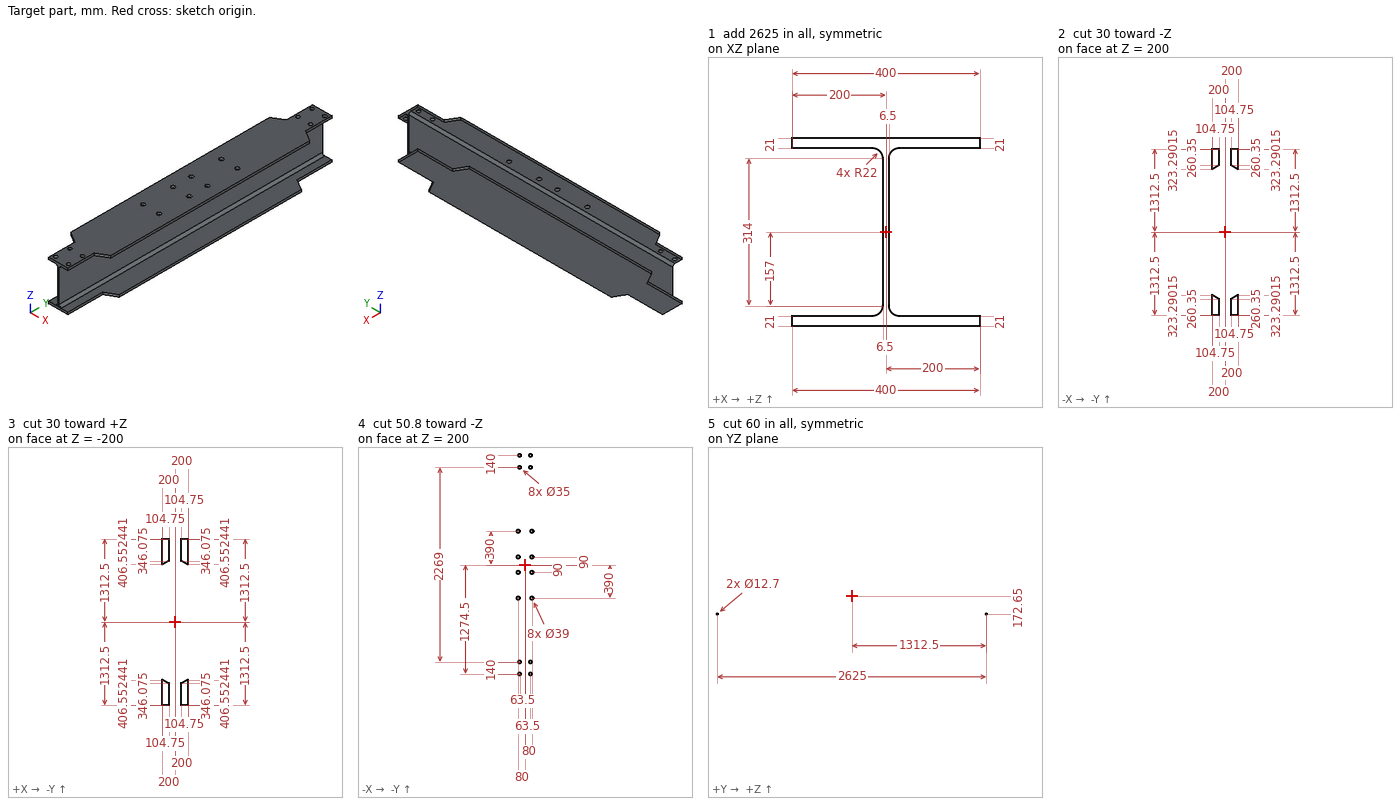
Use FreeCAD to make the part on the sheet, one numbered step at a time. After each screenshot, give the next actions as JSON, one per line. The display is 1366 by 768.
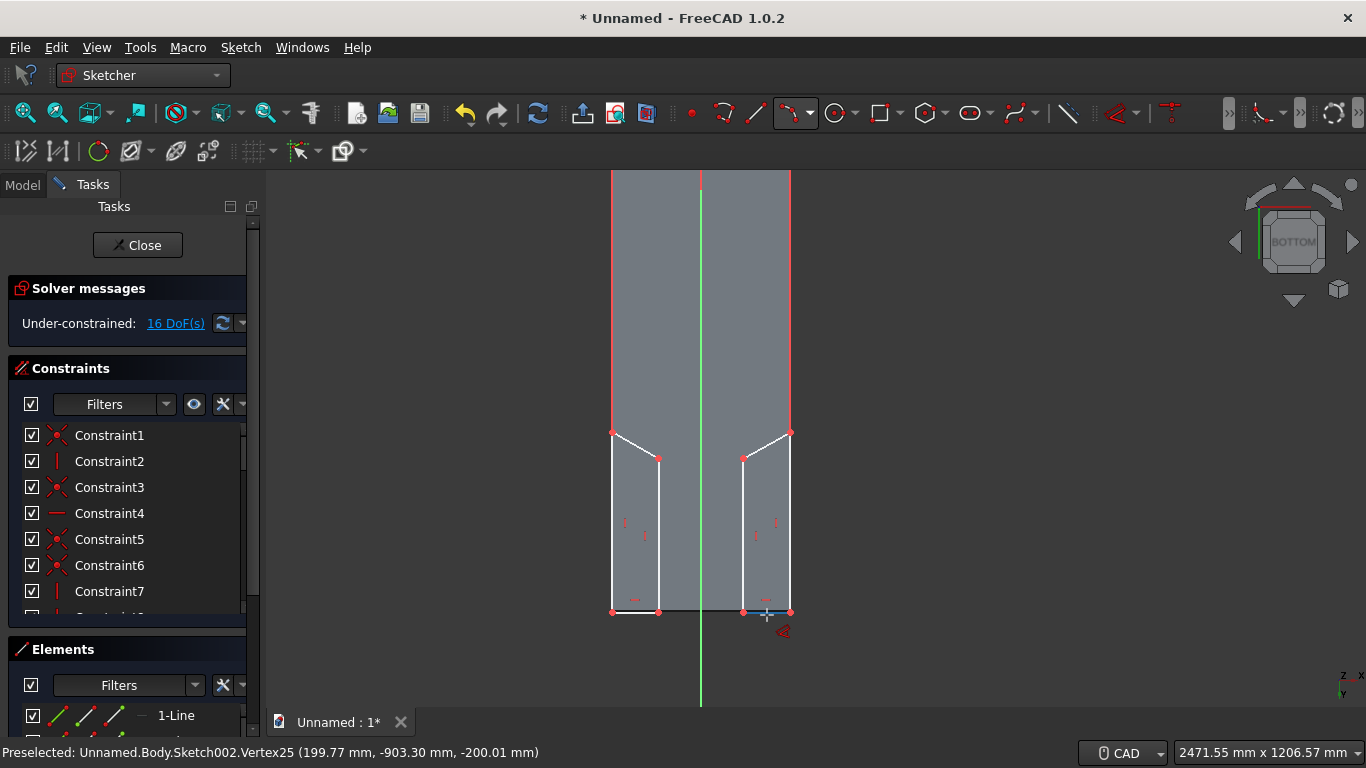
{"action": "left_click", "coordinate": [767, 613]}
{"action": "left_click", "coordinate": [767, 647]}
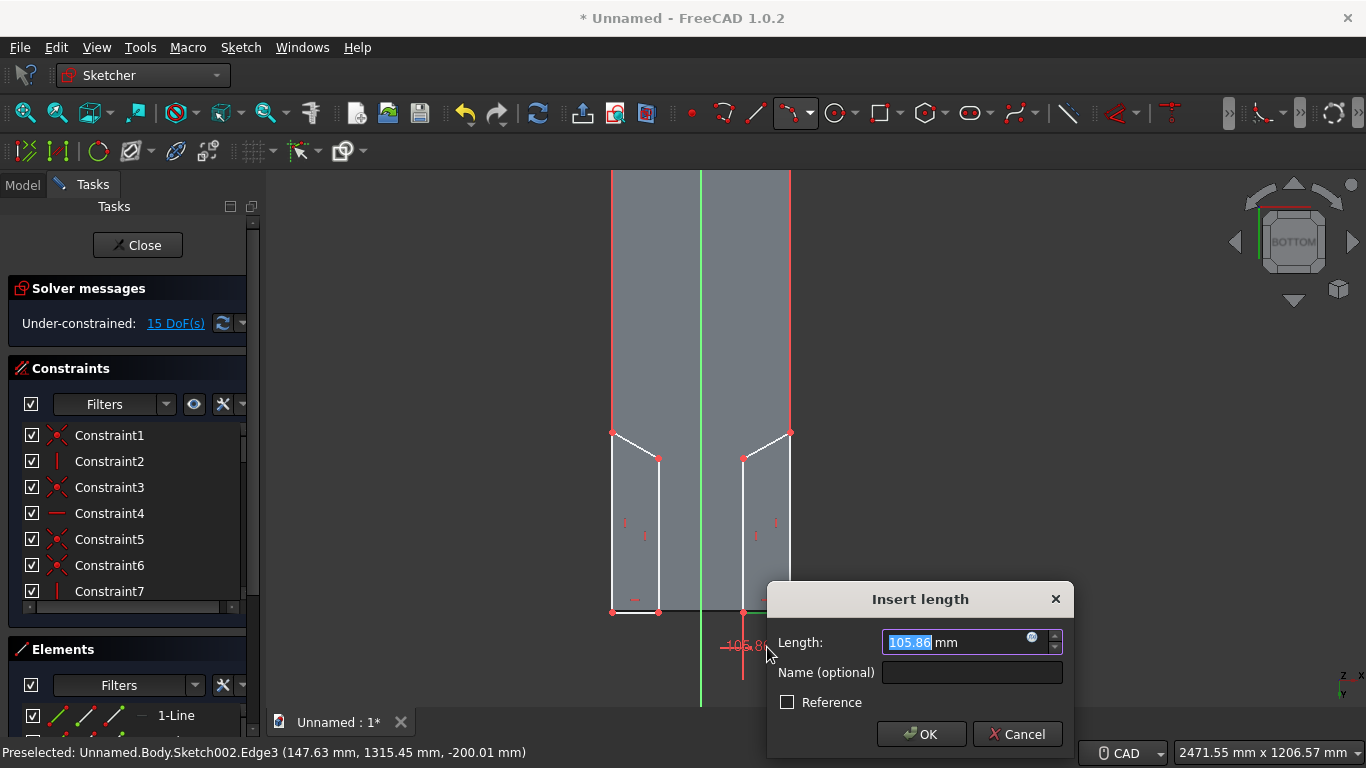
{"action": "type", "text": "104.75"}
{"action": "key", "text": "Return"}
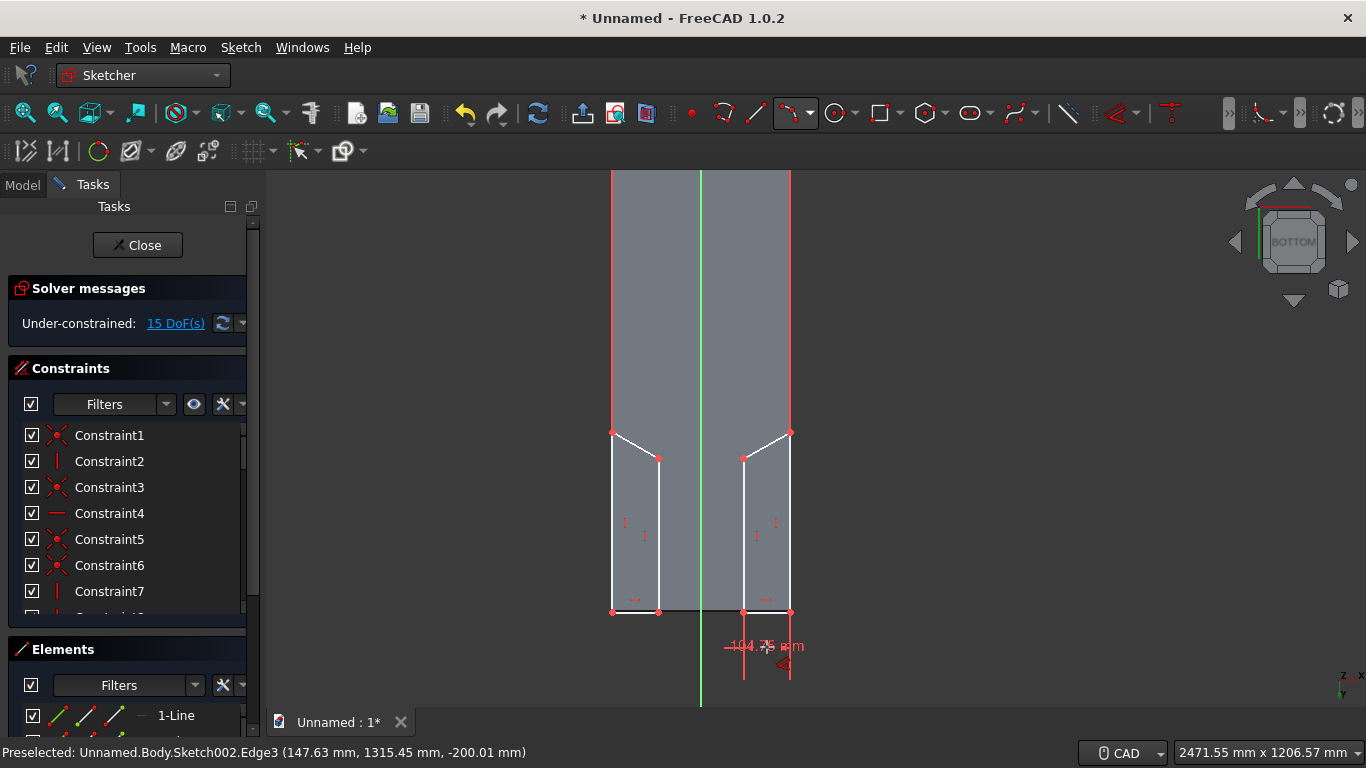
{"action": "left_click", "coordinate": [626, 613]}
{"action": "left_click", "coordinate": [636, 647]}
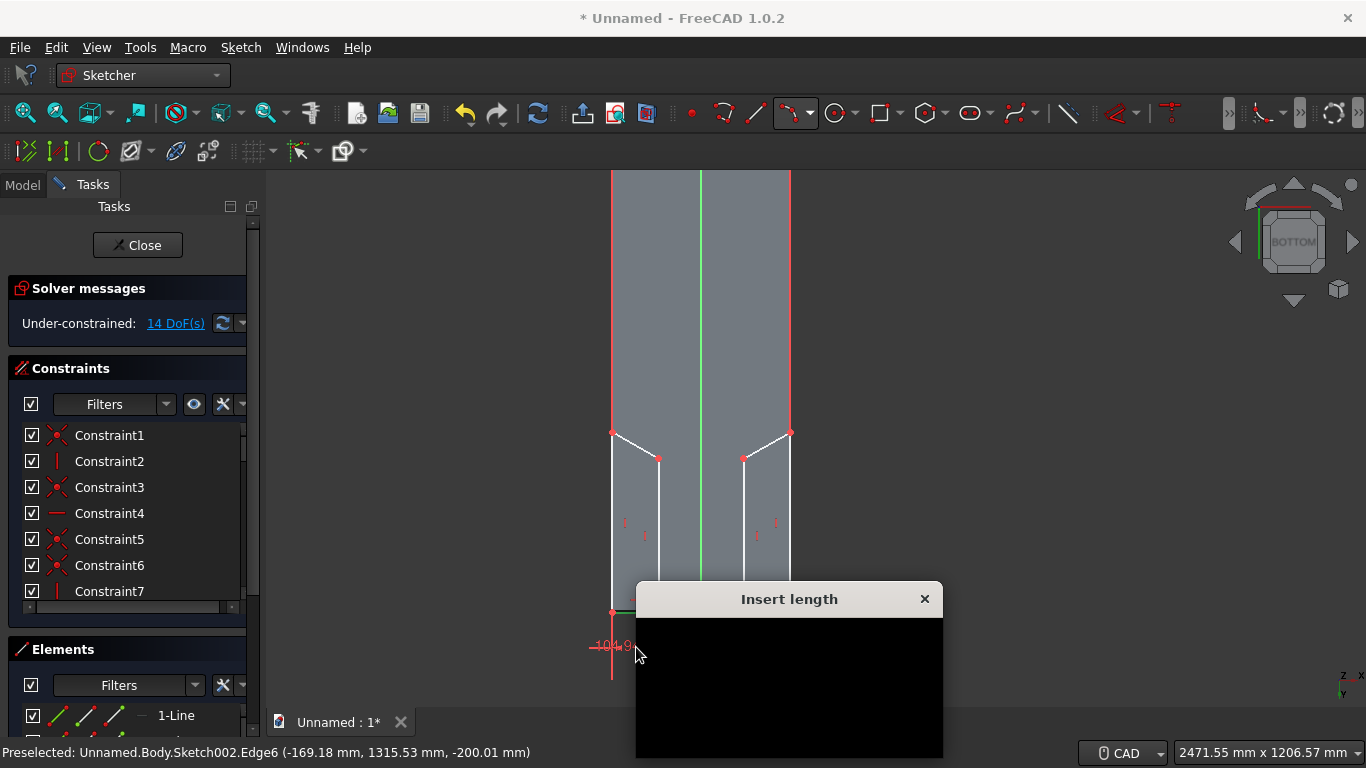
{"action": "type", "text": "104.75"}
{"action": "key", "text": "Return"}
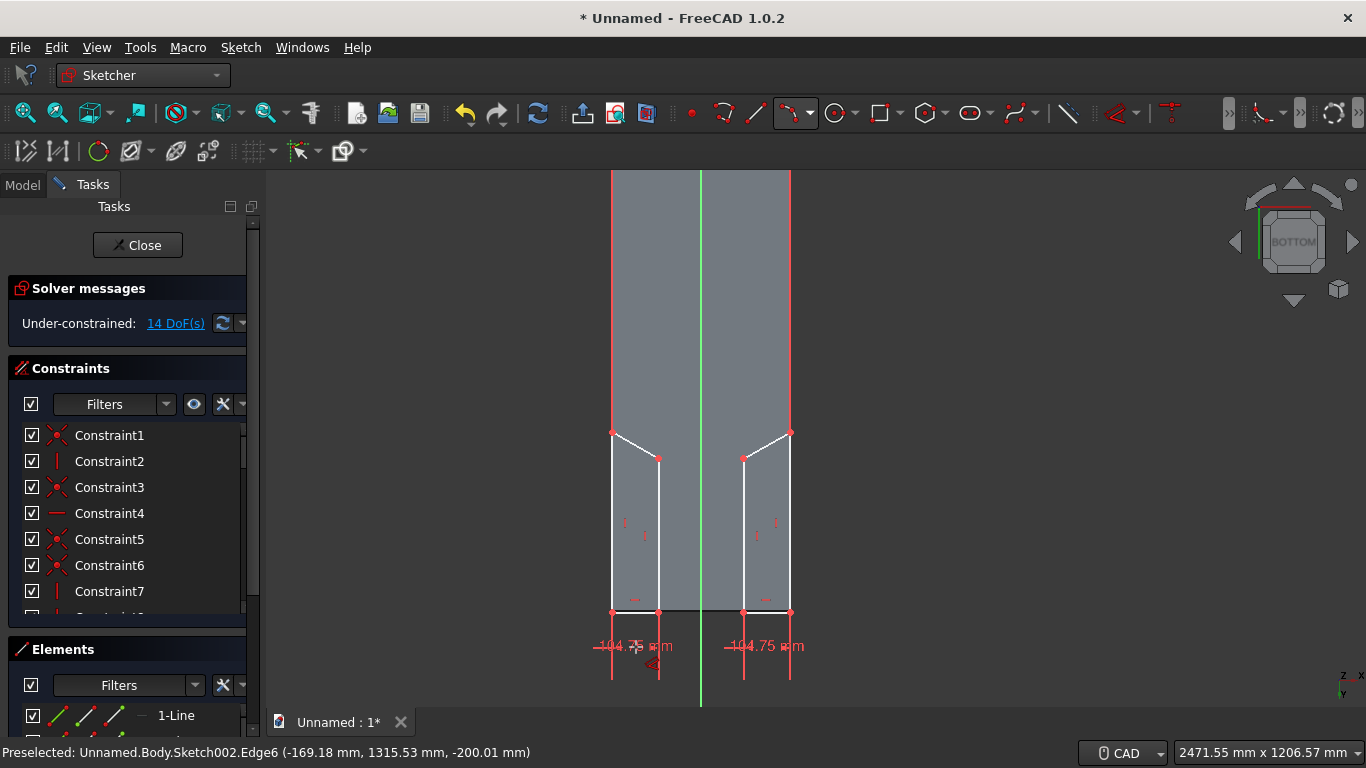
{"action": "scroll", "coordinate": [767, 616], "scroll_direction": "down", "scroll_amount": 6}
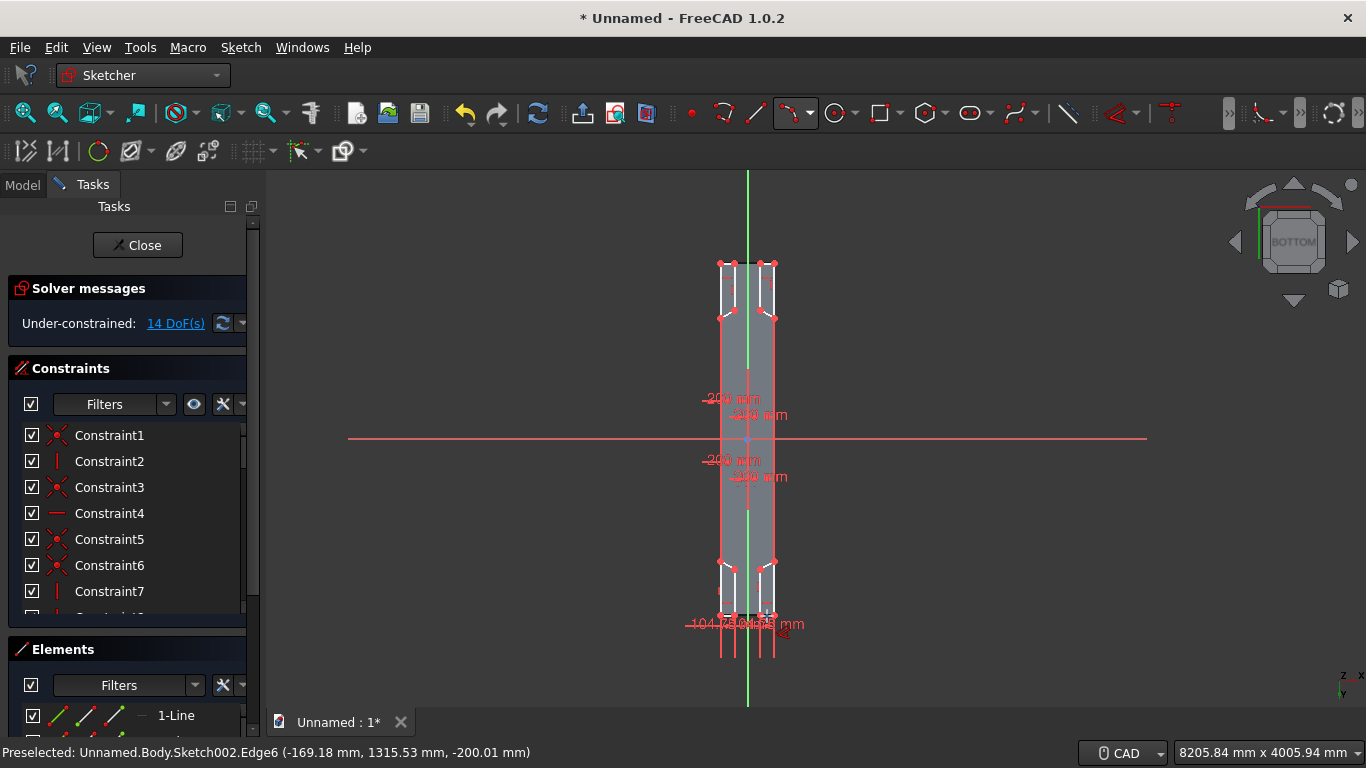
{"action": "scroll", "coordinate": [731, 264], "scroll_direction": "up", "scroll_amount": 6}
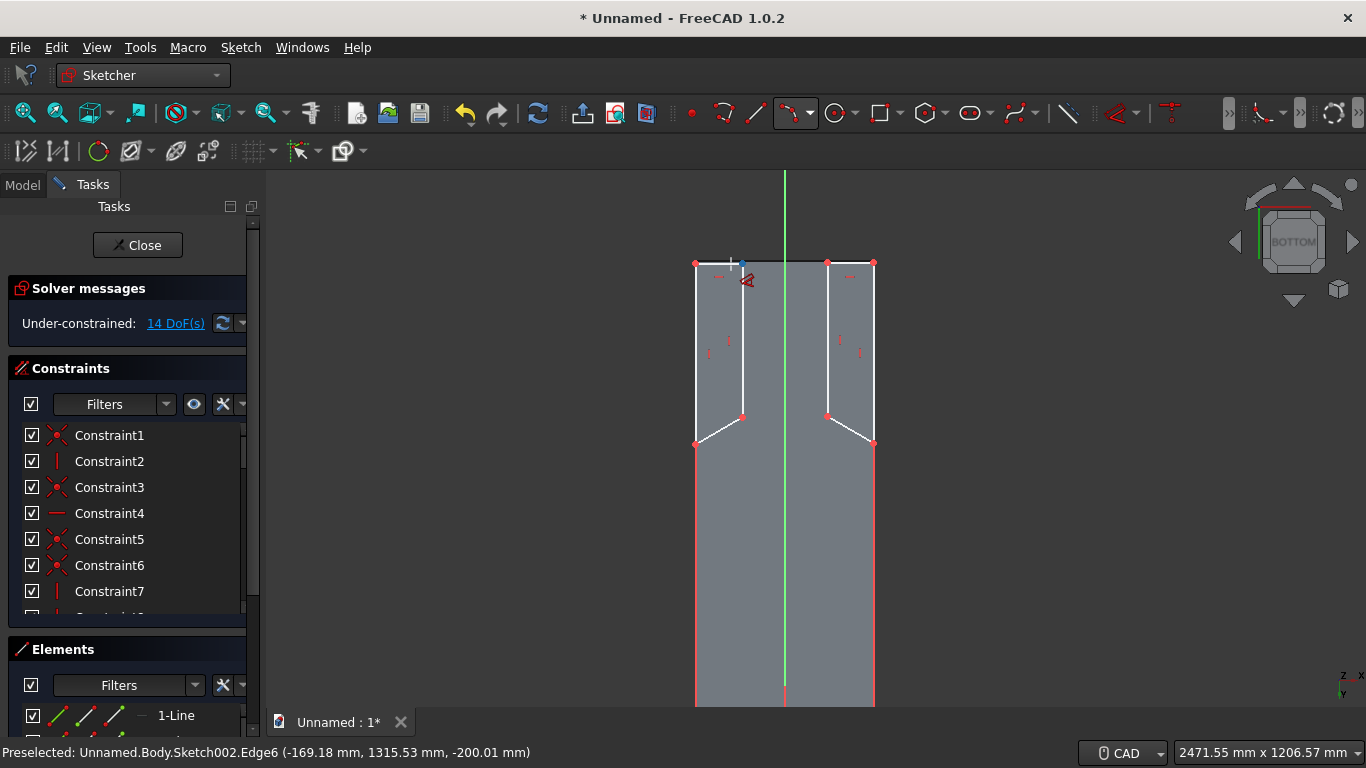
{"action": "left_click", "coordinate": [729, 264]}
{"action": "left_click", "coordinate": [719, 230]}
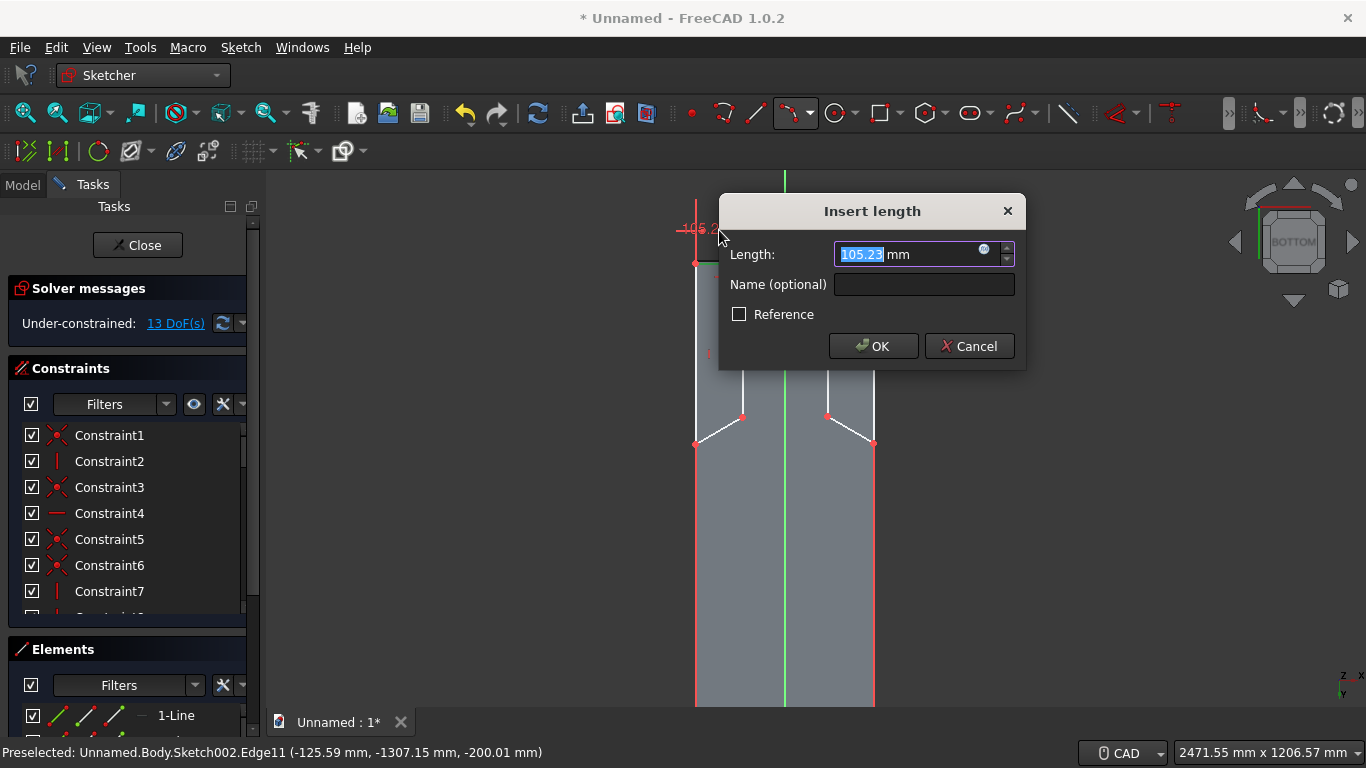
{"action": "type", "text": "104.75"}
{"action": "key", "text": "Return"}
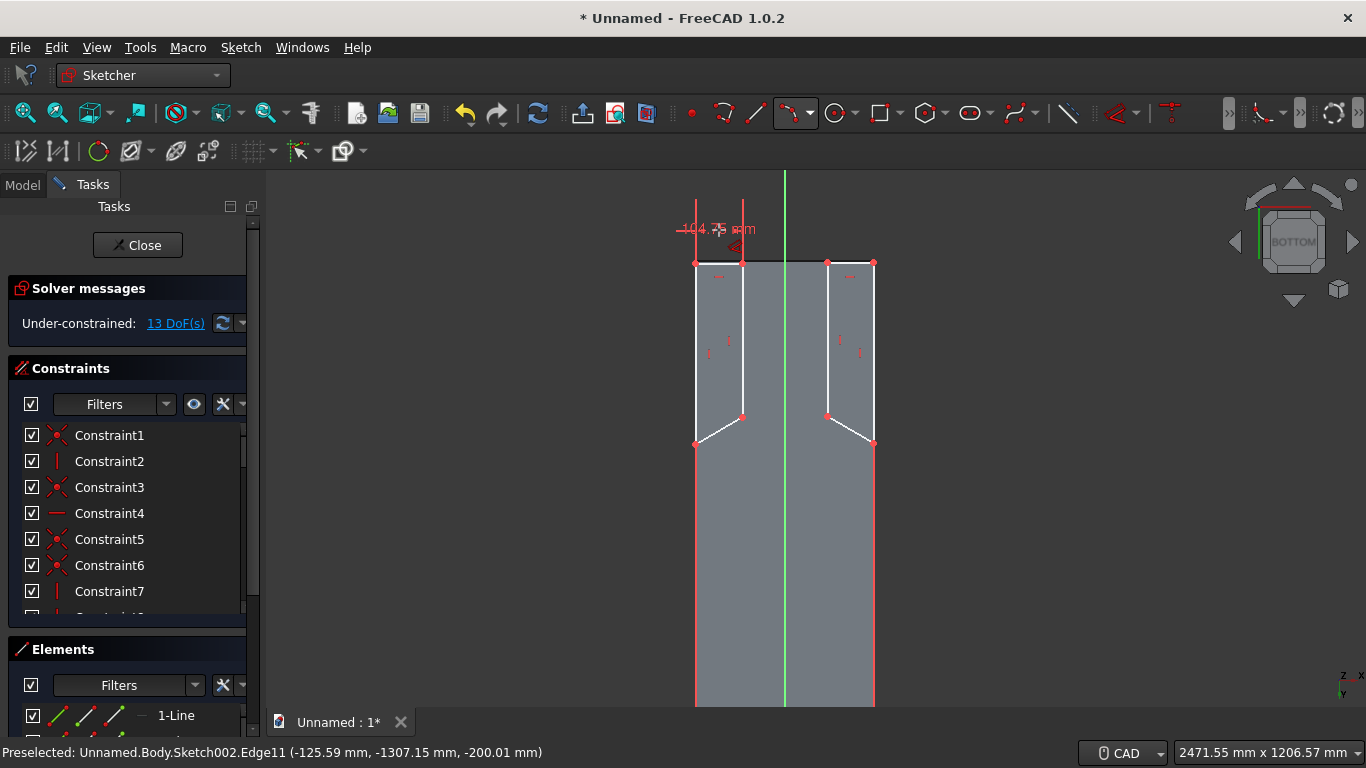
{"action": "left_click", "coordinate": [860, 263]}
{"action": "left_click", "coordinate": [851, 229]}